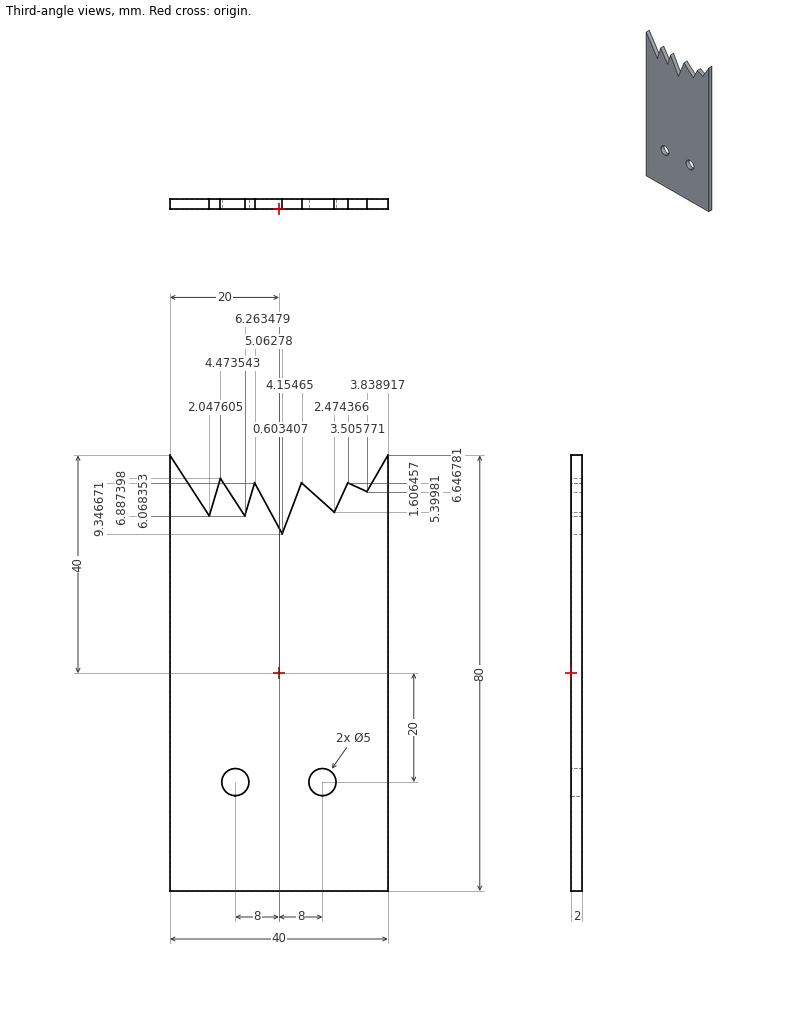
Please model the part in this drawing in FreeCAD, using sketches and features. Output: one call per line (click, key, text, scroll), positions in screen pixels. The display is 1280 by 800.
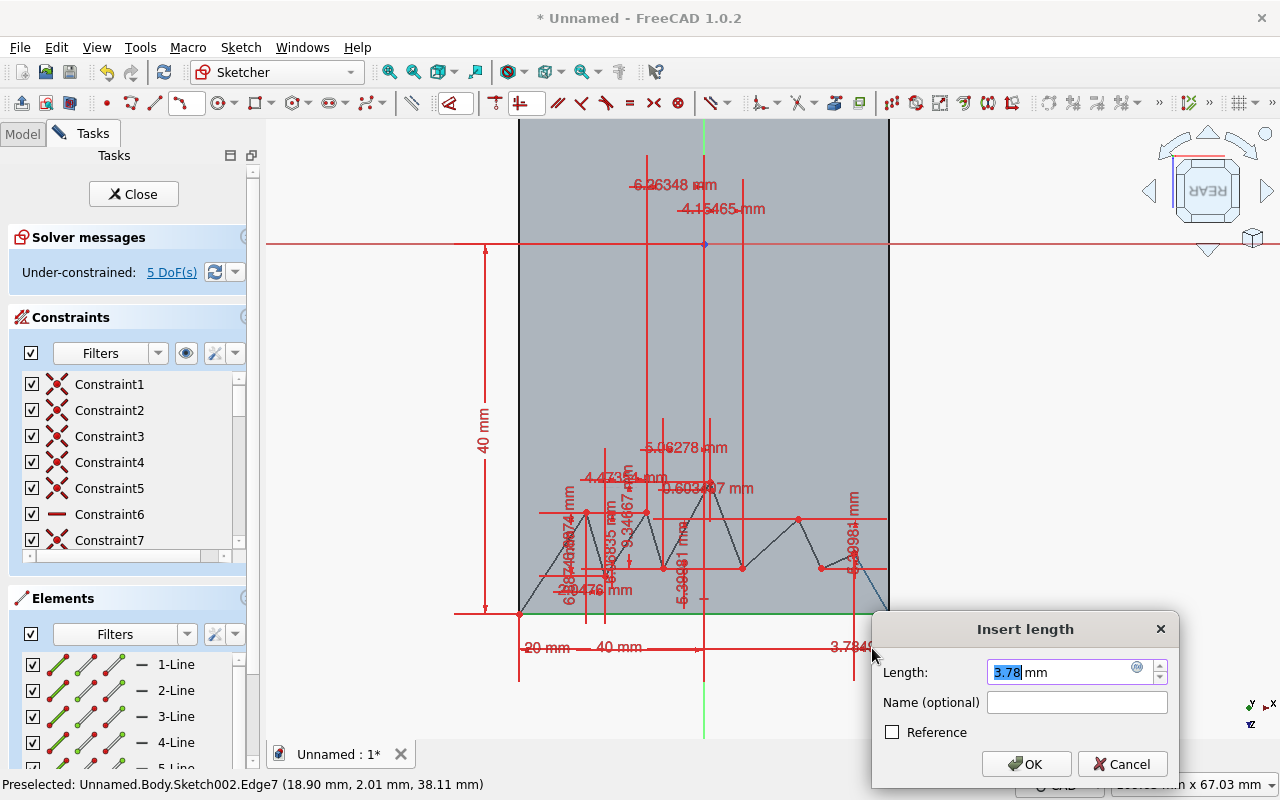
text(3.838917)
key(Return)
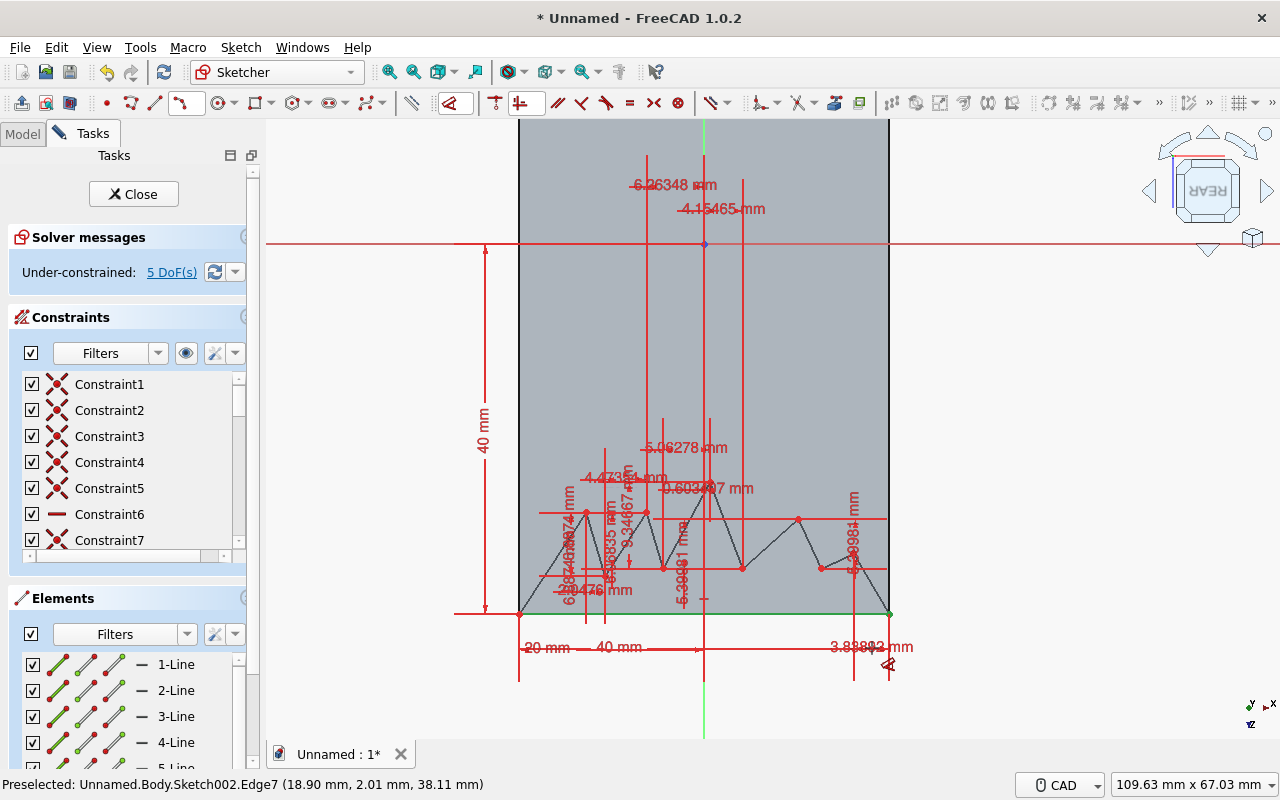
click(879, 596)
click(923, 584)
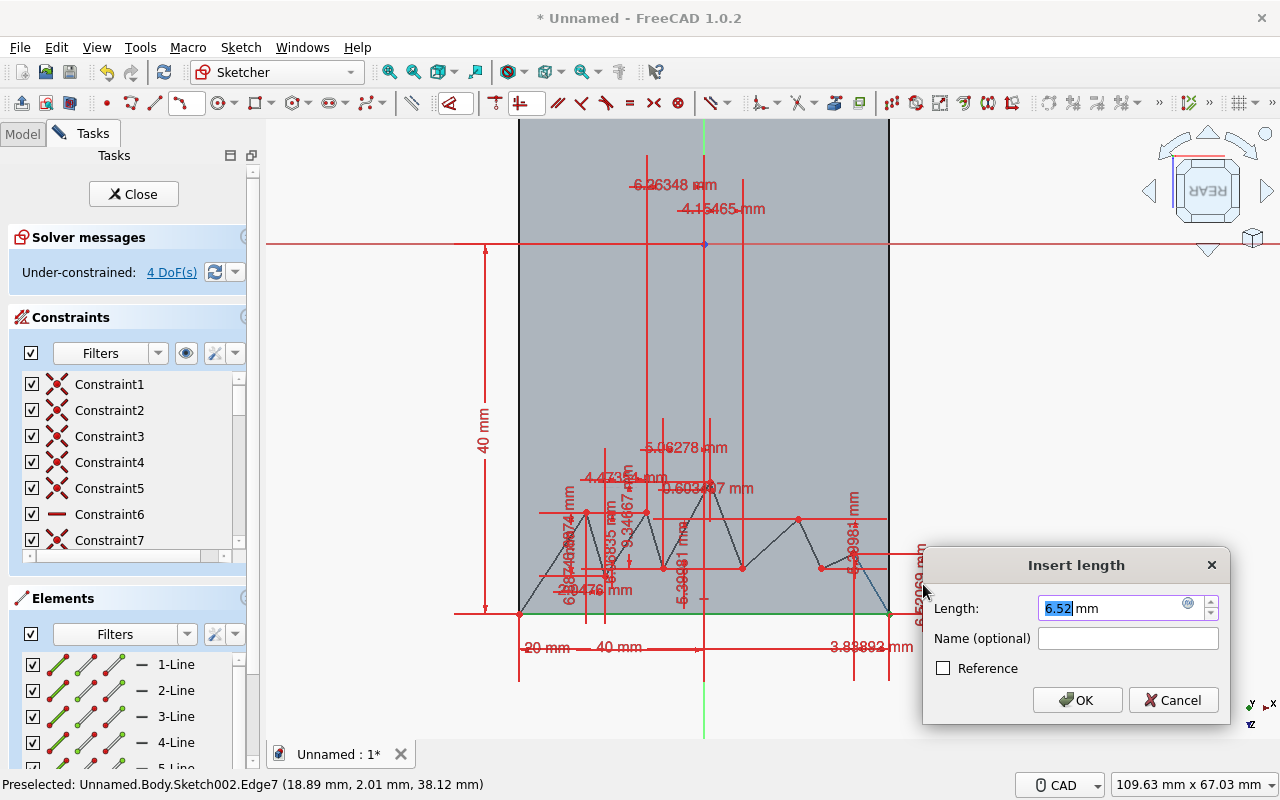
text(6.646781)
key(Return)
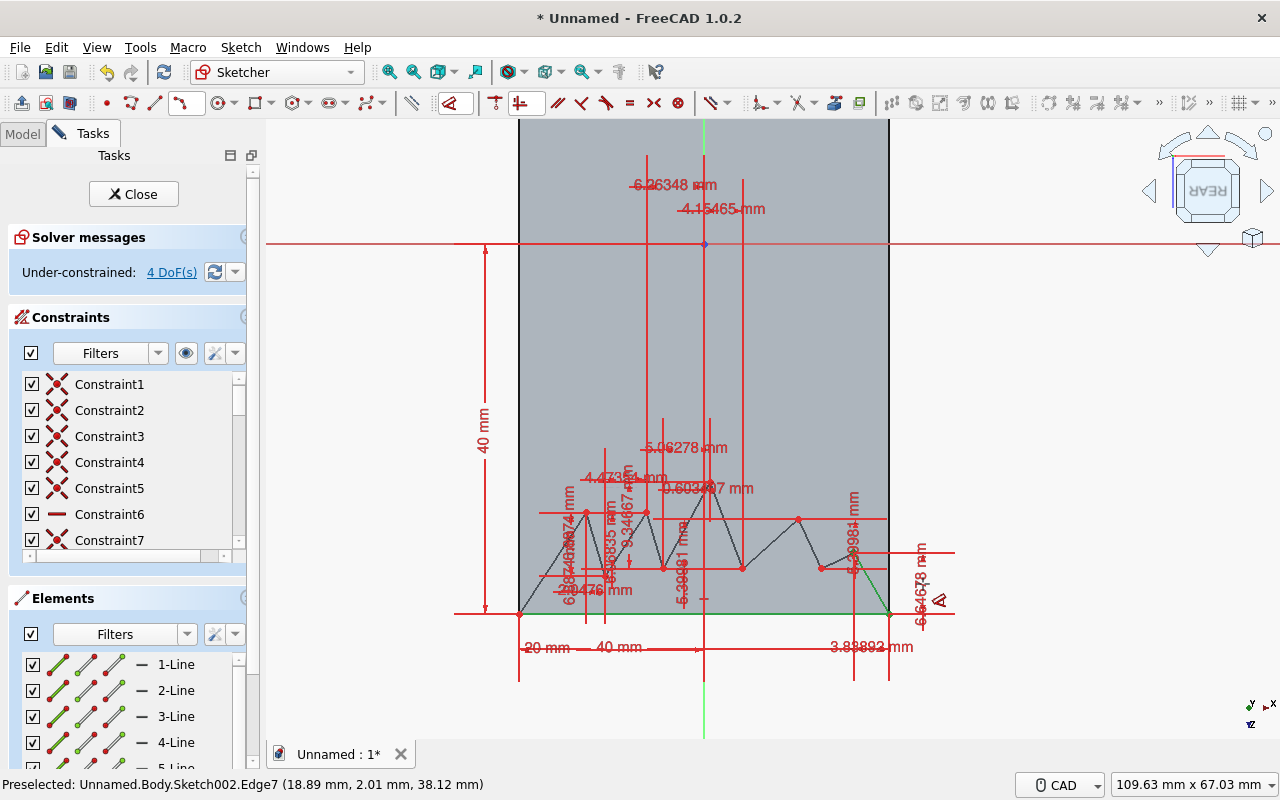
scroll(844, 558, up, 2)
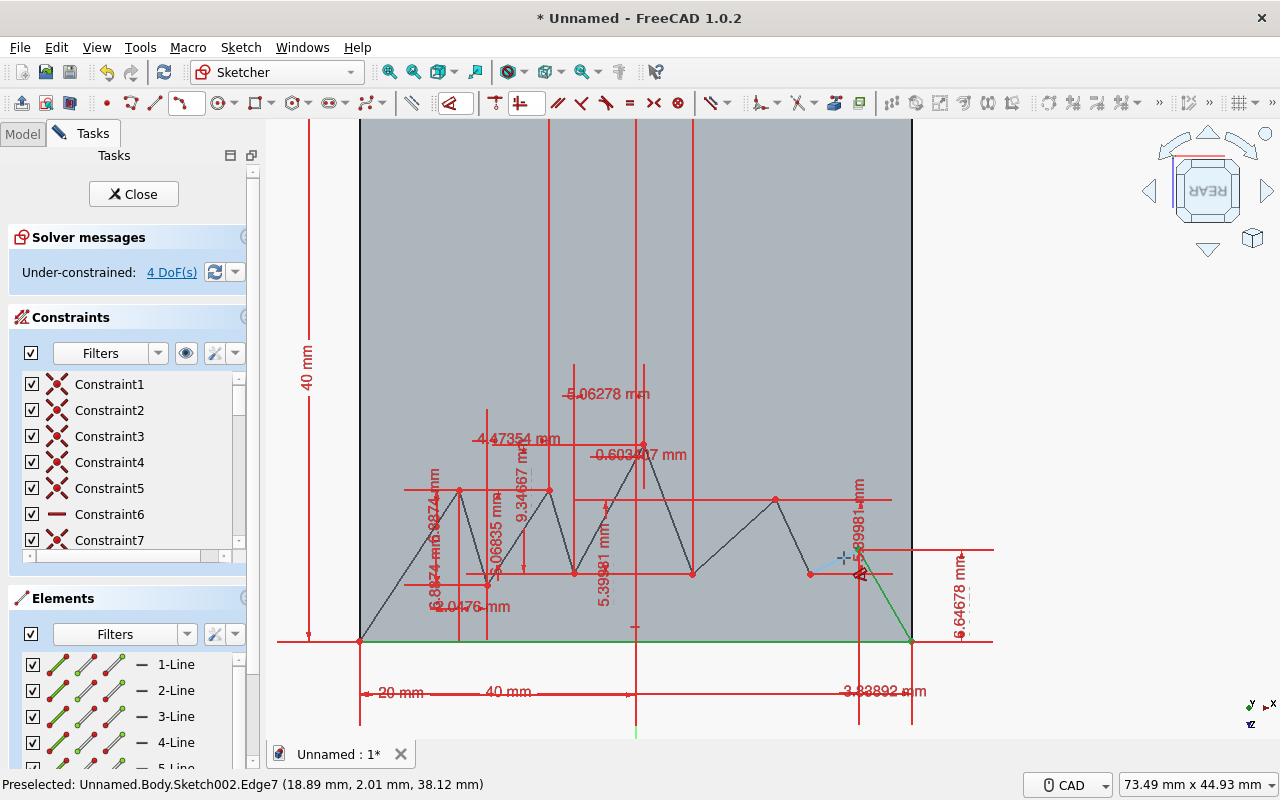
click(844, 557)
click(834, 608)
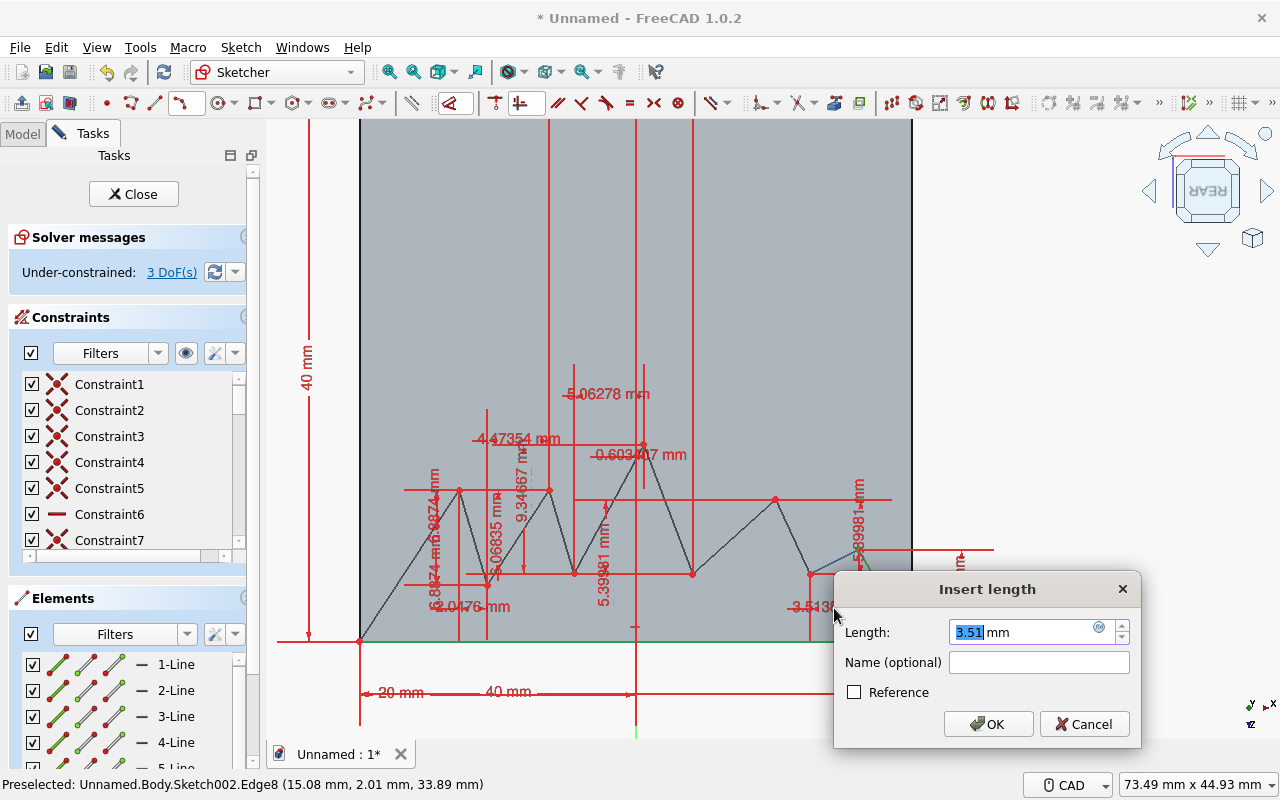
text(3.505771)
key(Return)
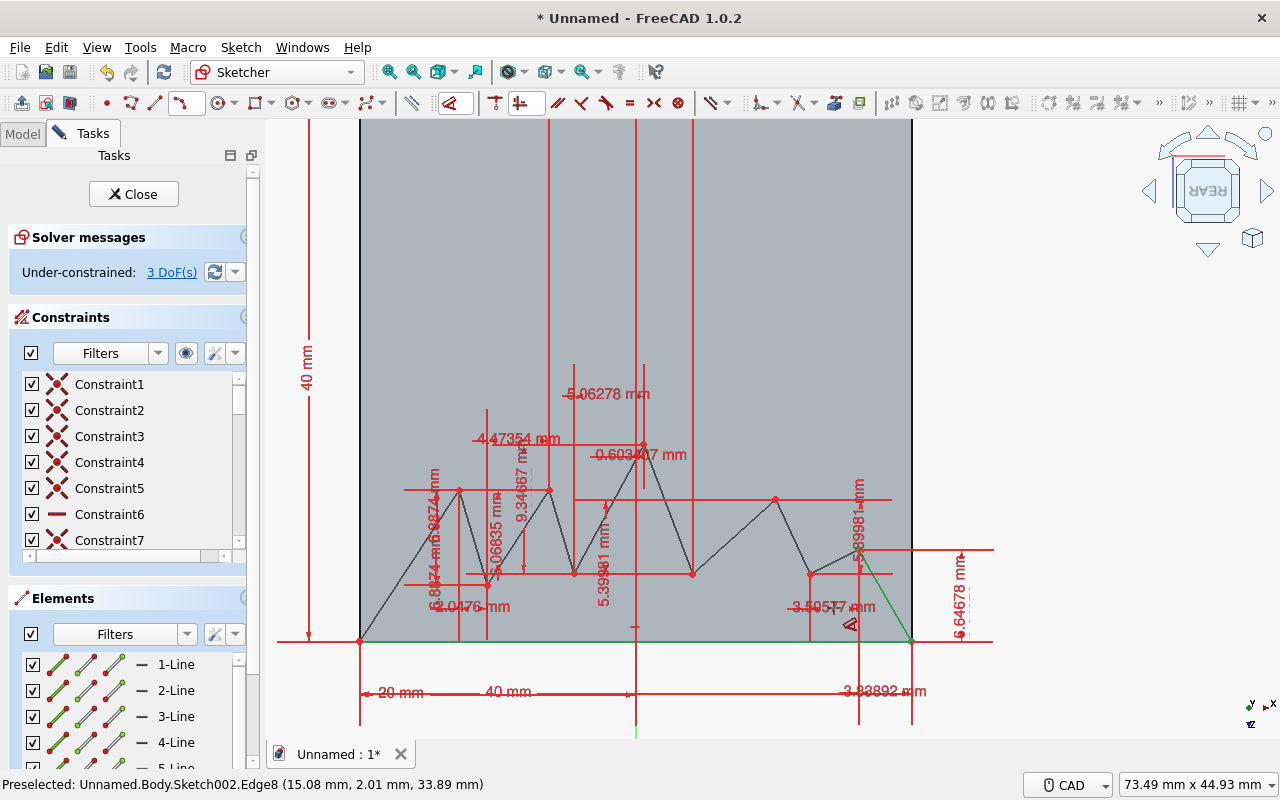
scroll(844, 557, up, 3)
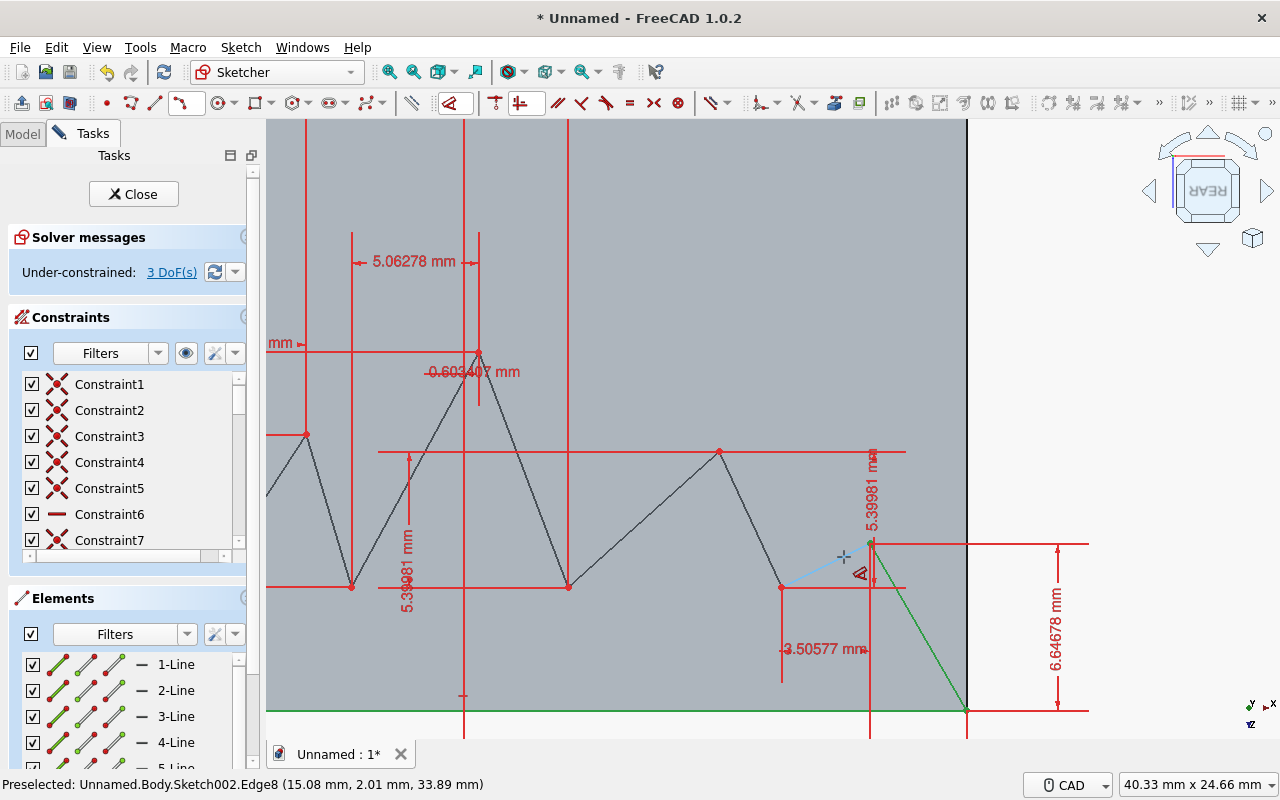
click(844, 557)
click(904, 566)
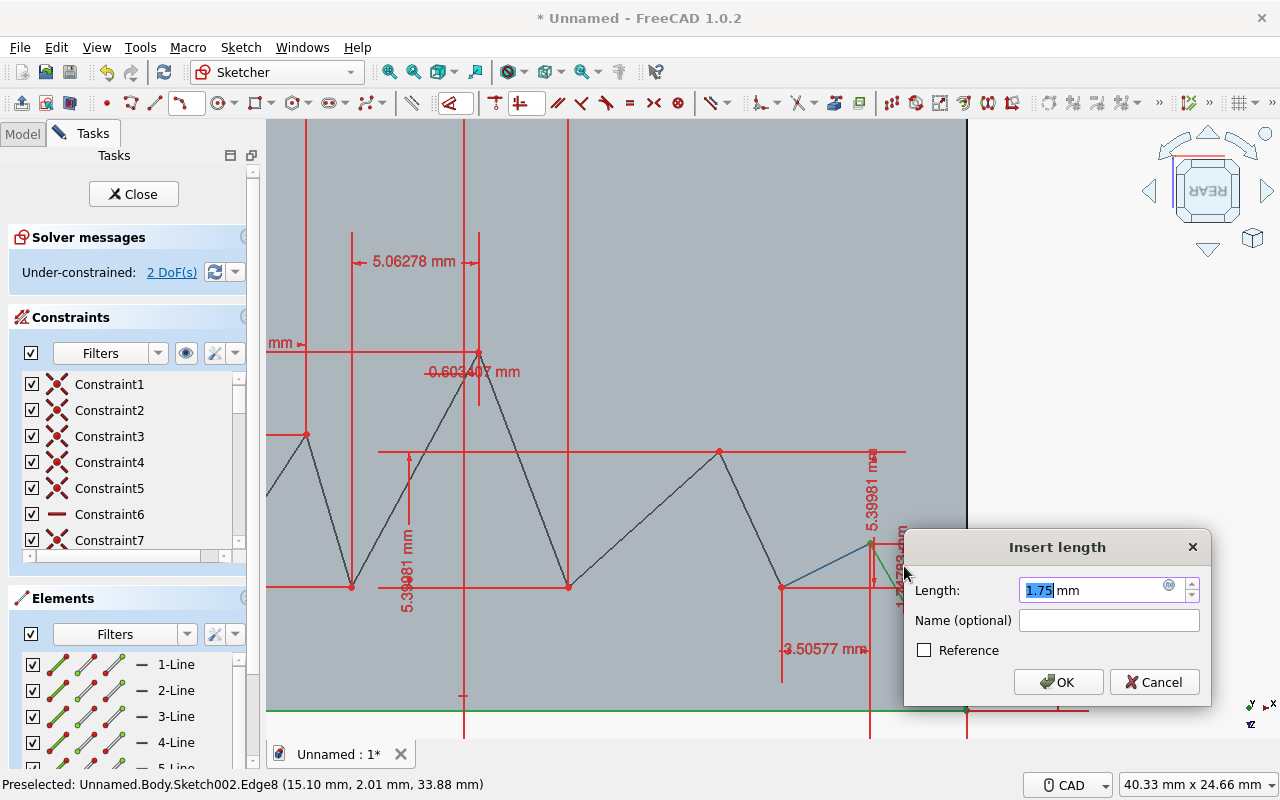
text(1.606457)
key(Return)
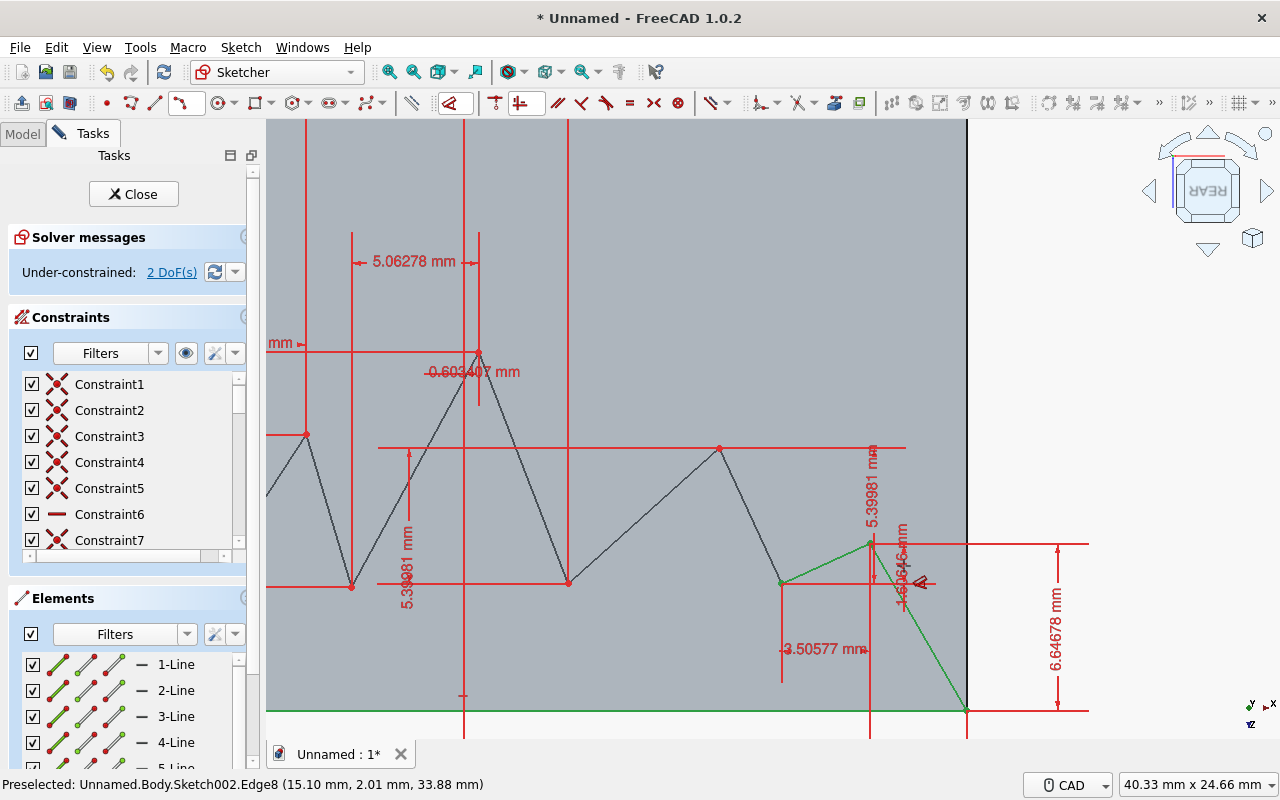
click(763, 543)
click(751, 618)